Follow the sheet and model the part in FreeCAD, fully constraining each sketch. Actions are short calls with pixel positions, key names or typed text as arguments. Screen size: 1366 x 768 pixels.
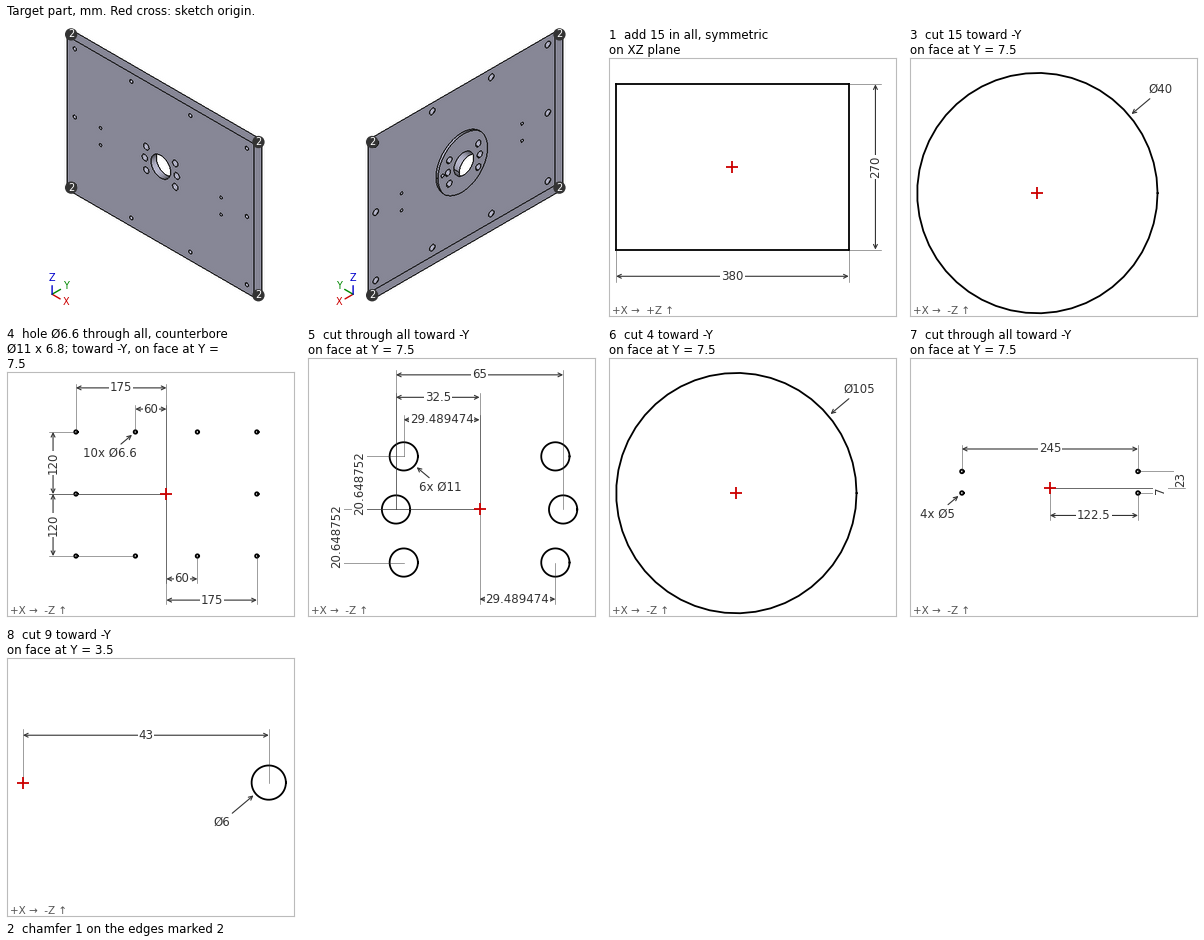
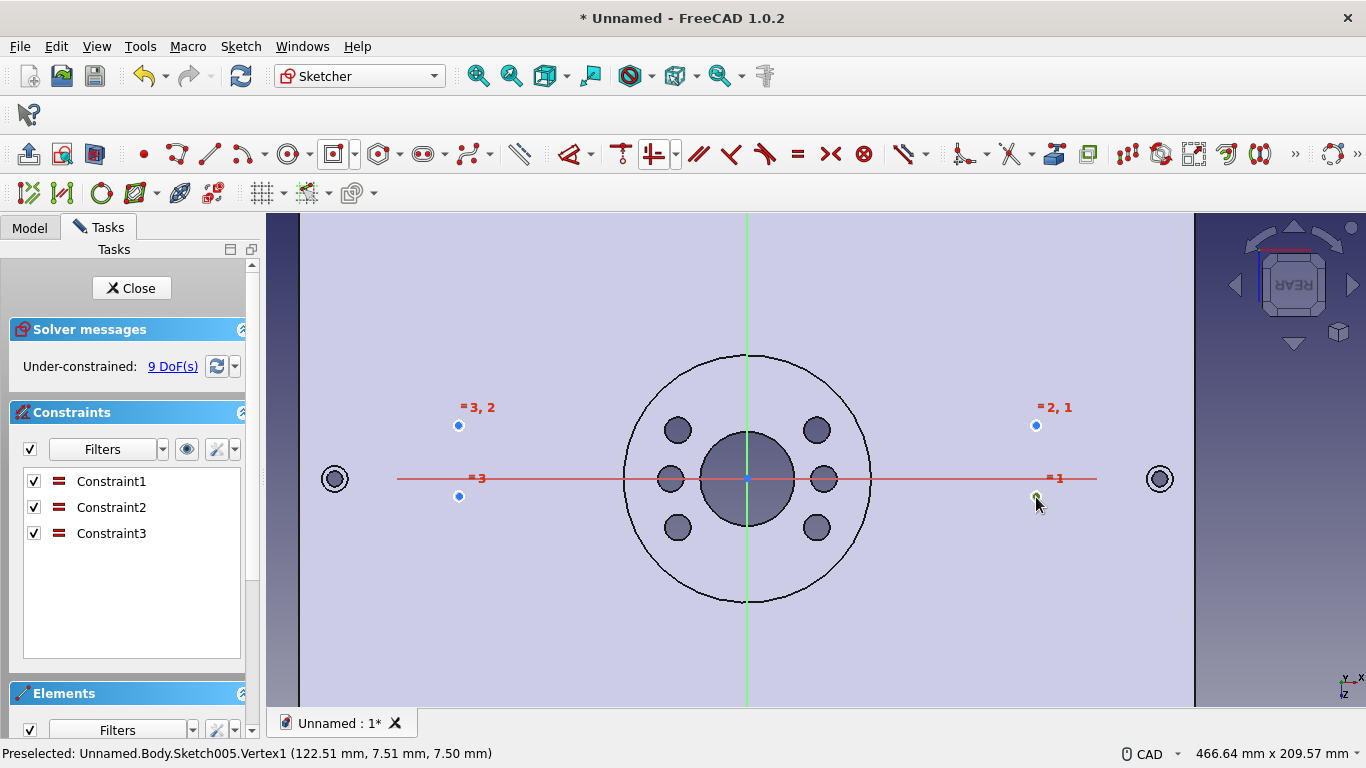
click(1036, 426)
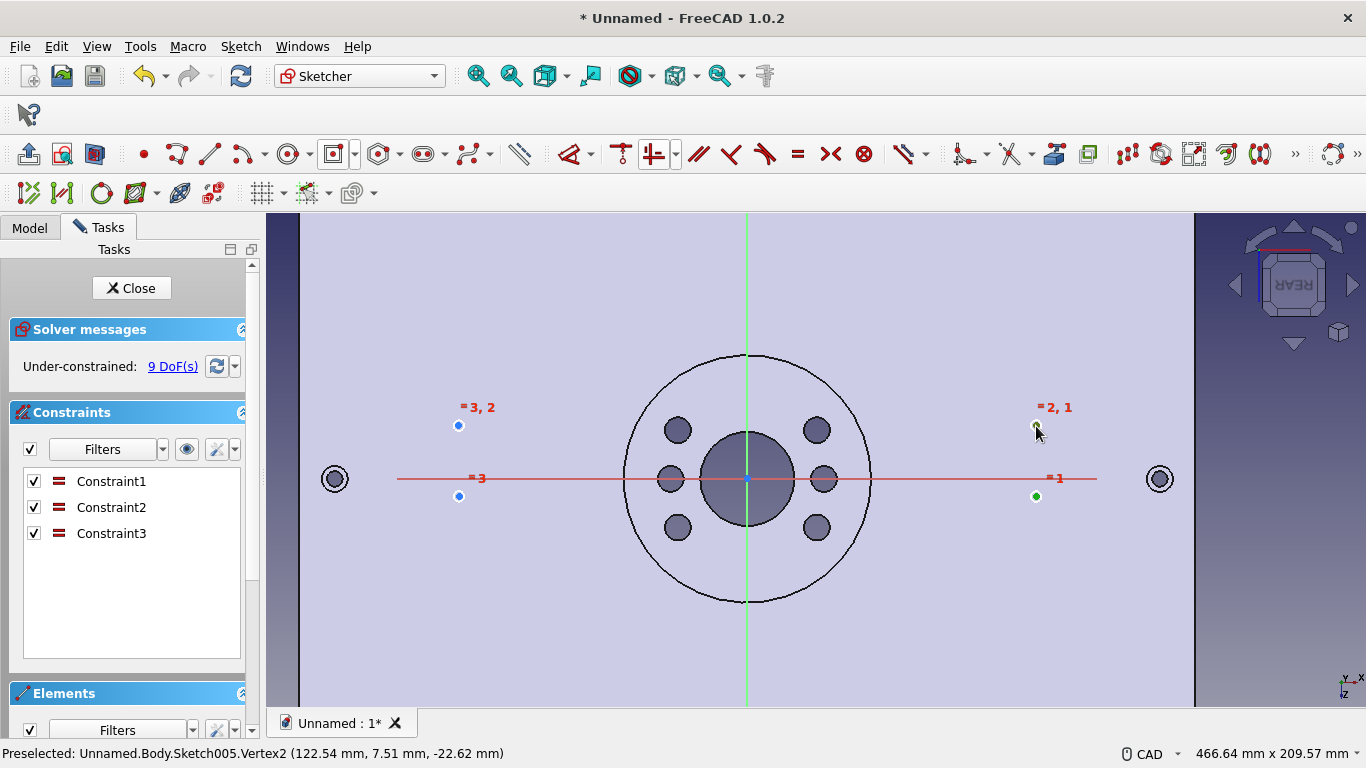
key(v)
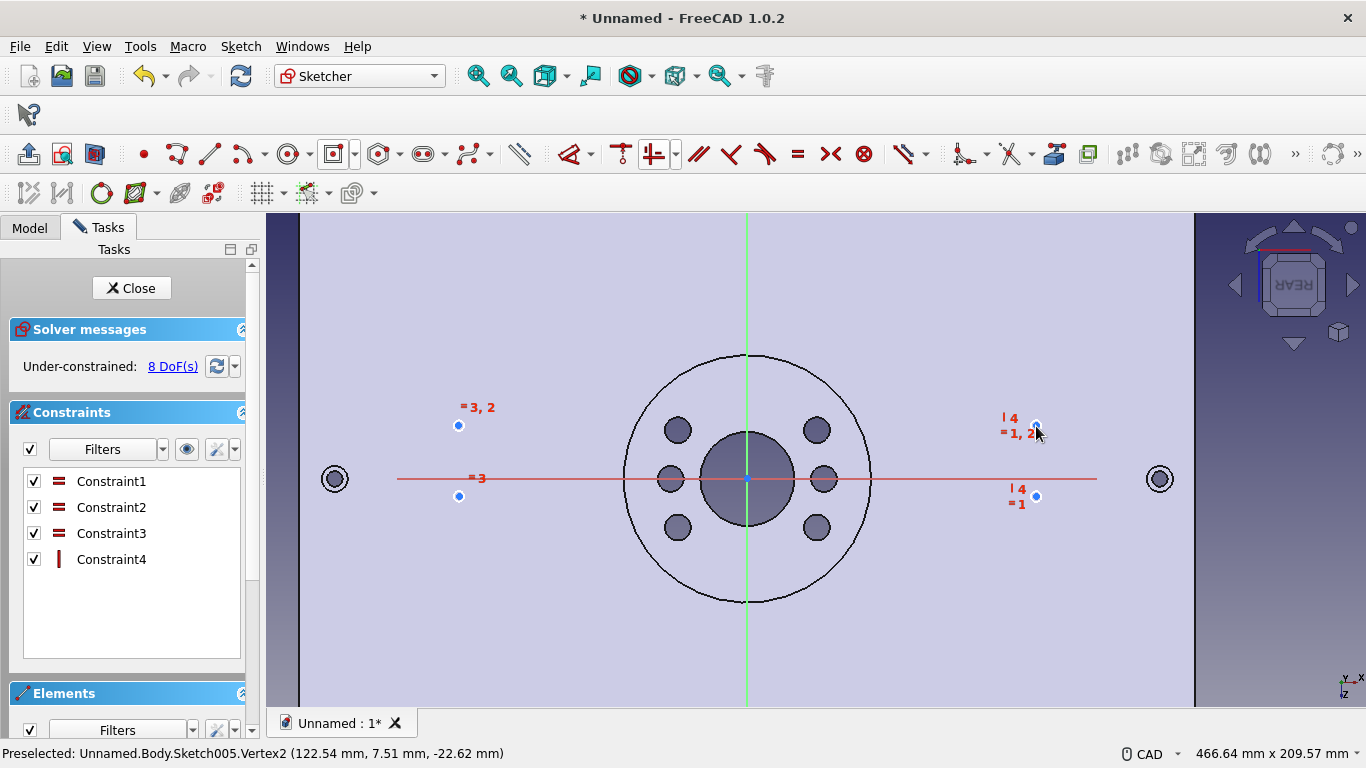
click(1036, 426)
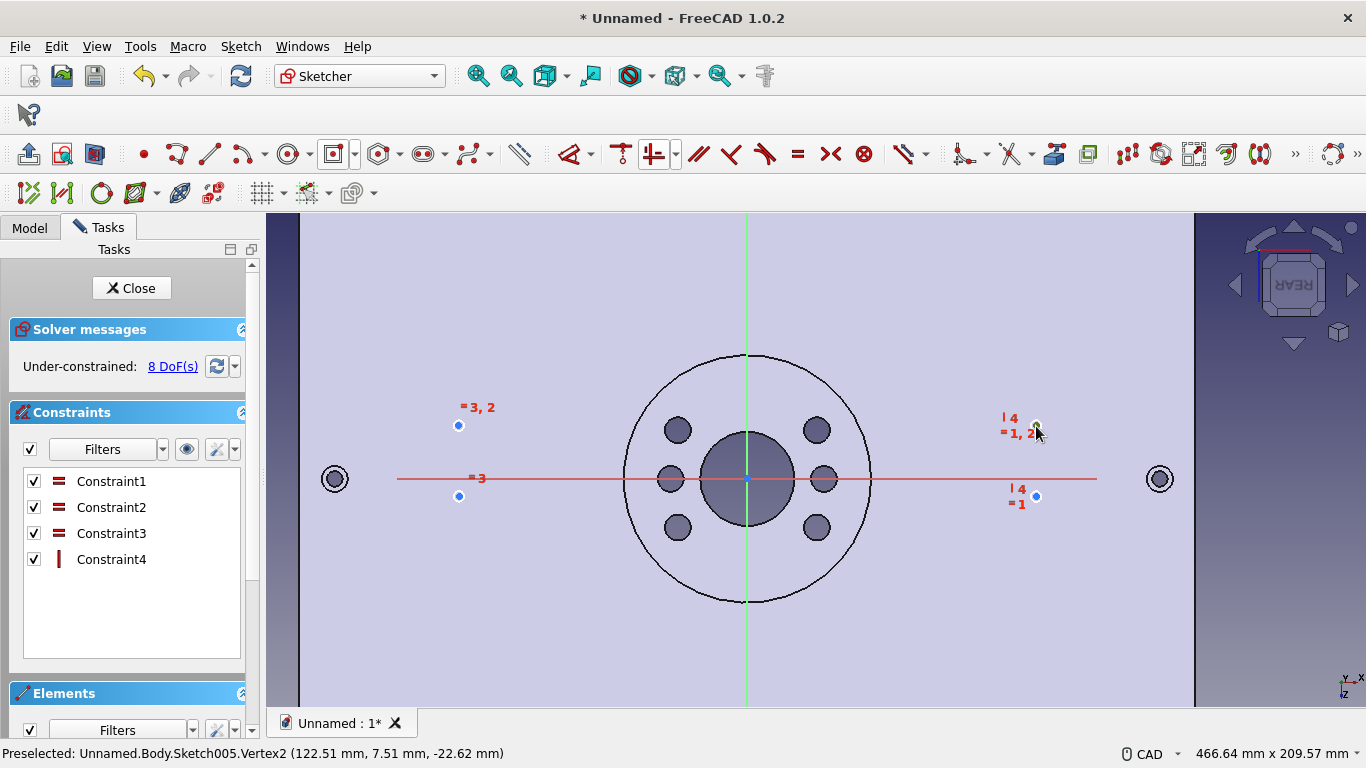
click(459, 426)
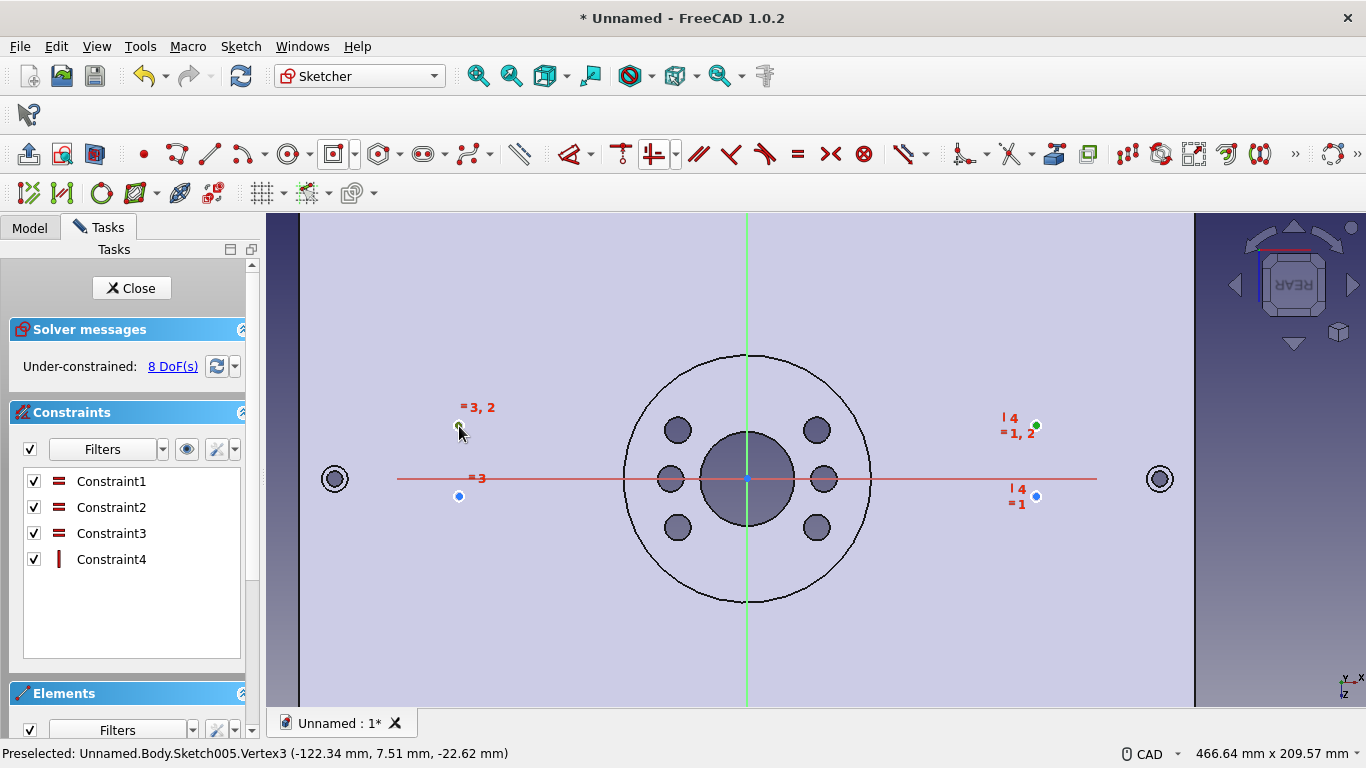
key(h)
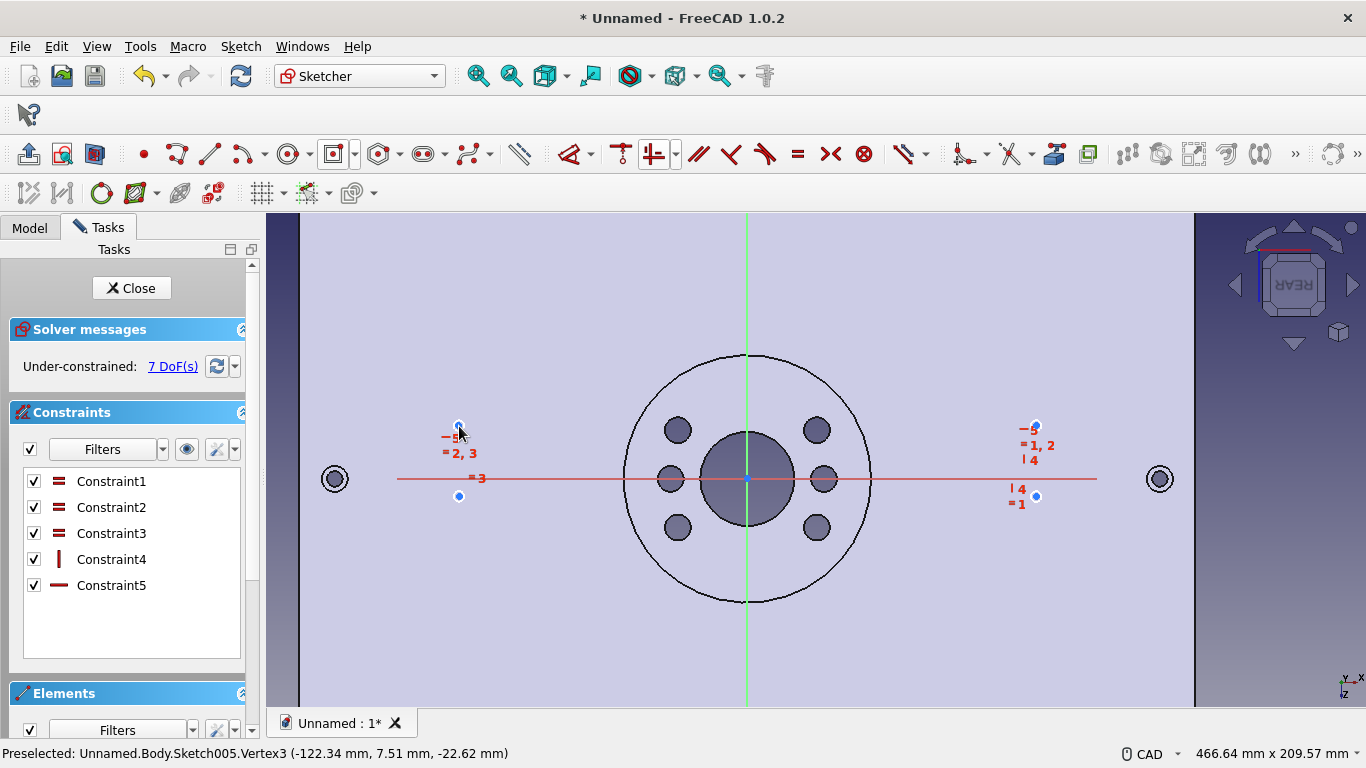
click(459, 426)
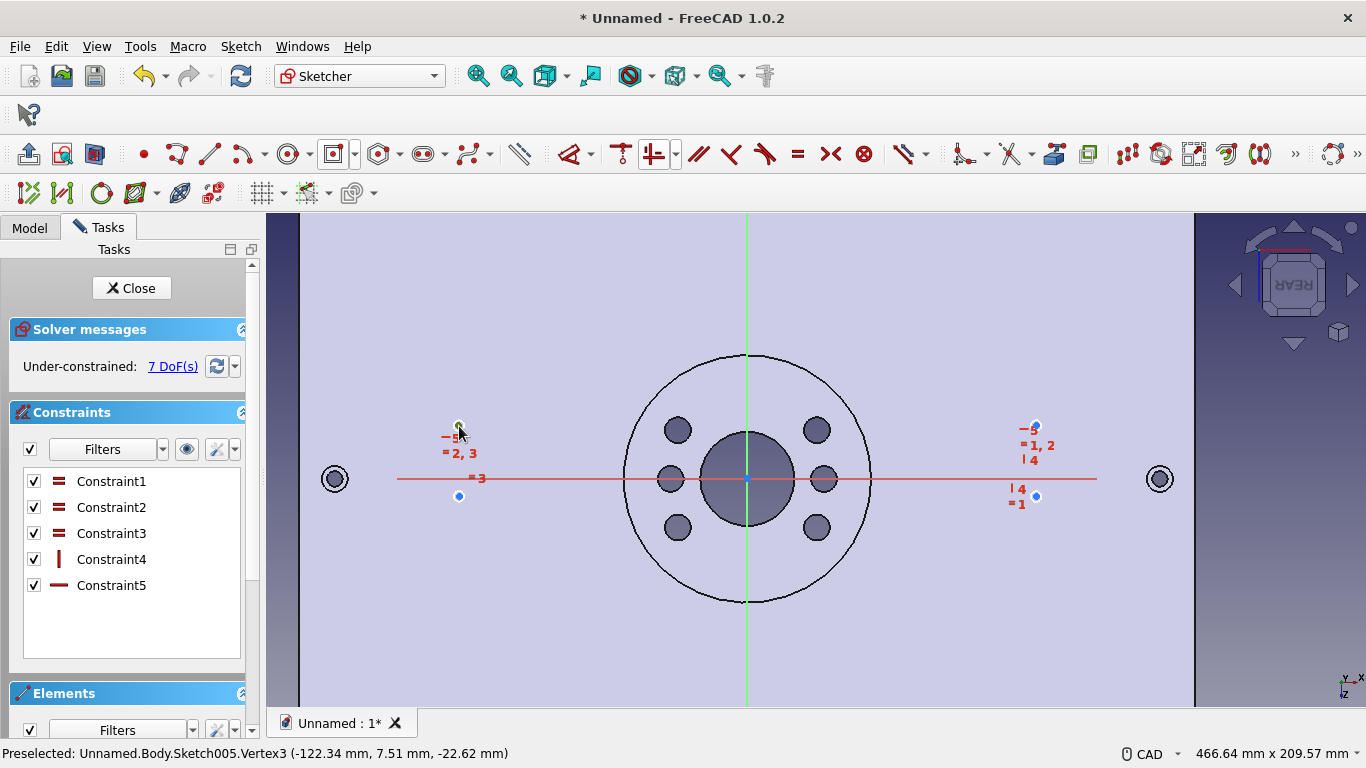
click(459, 496)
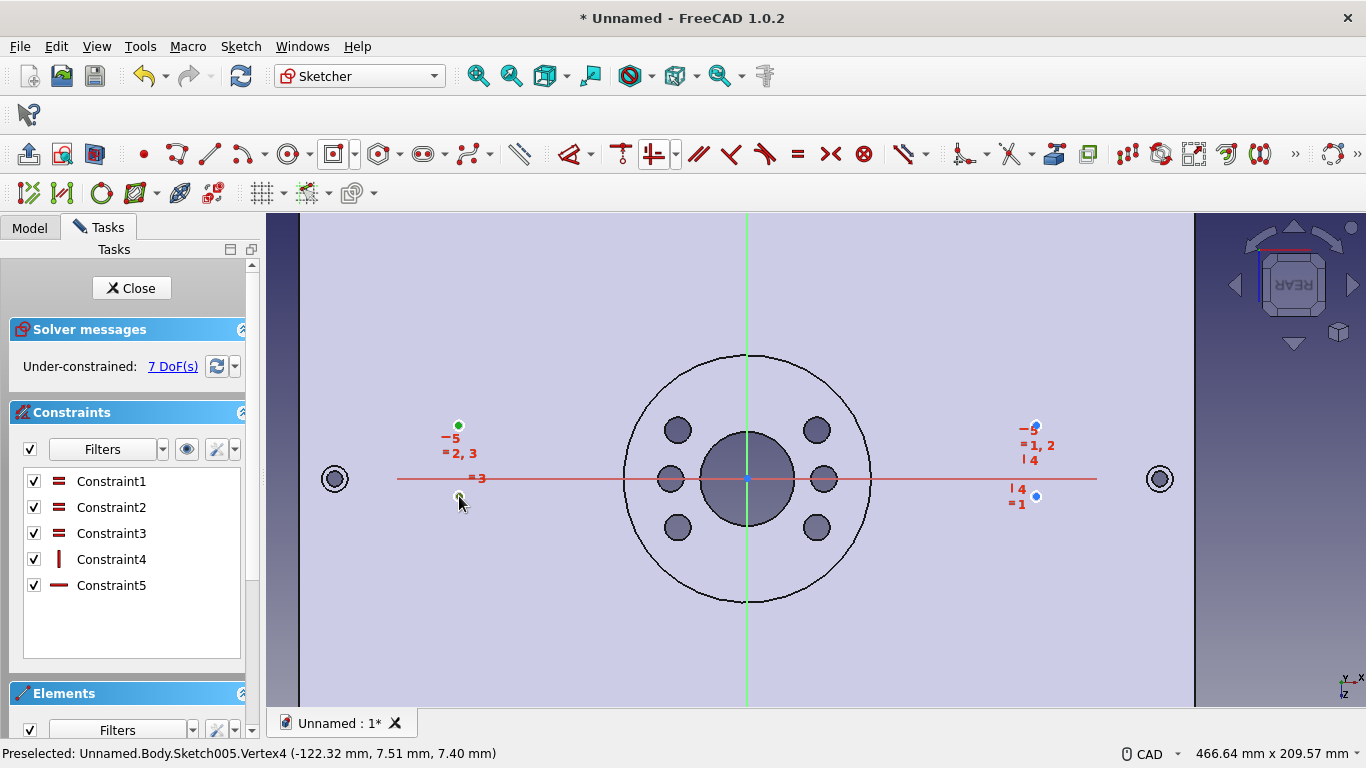
click(676, 154)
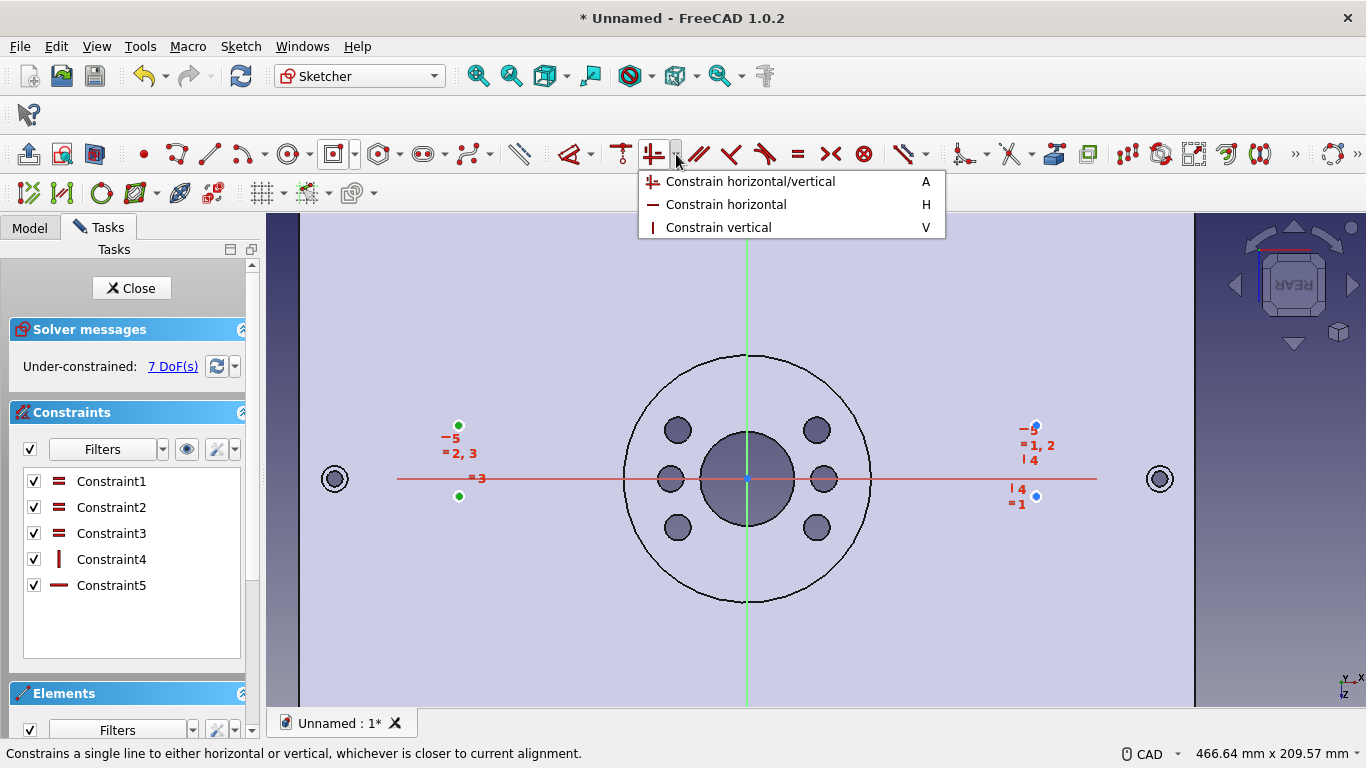
click(792, 228)